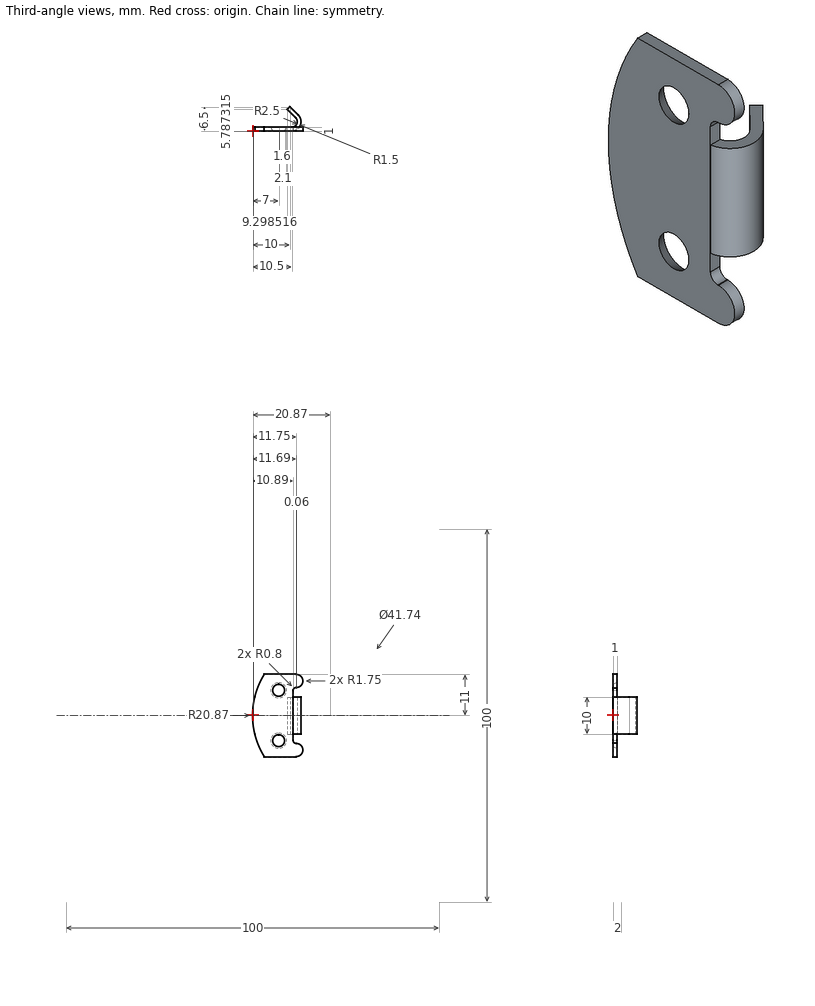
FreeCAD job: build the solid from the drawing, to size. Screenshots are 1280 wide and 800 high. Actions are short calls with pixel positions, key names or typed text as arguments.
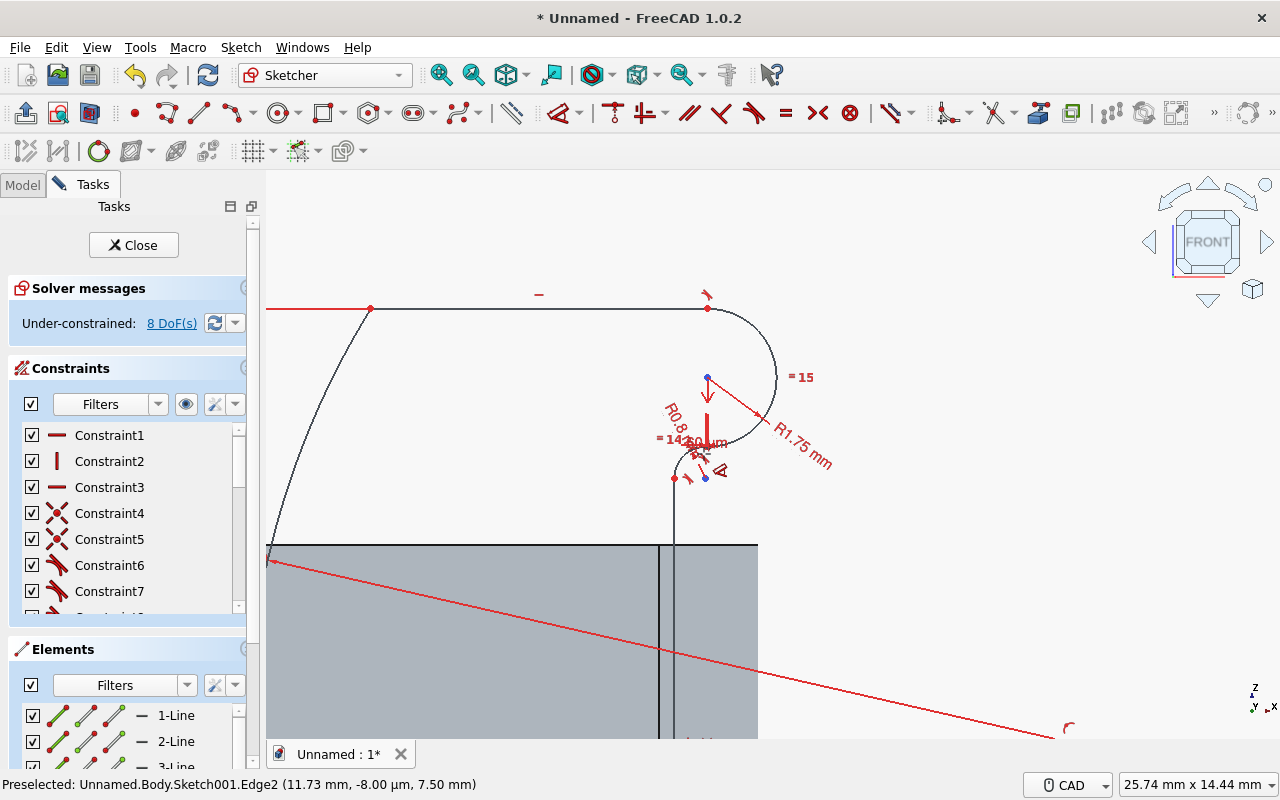
scroll(862, 220, down, 4)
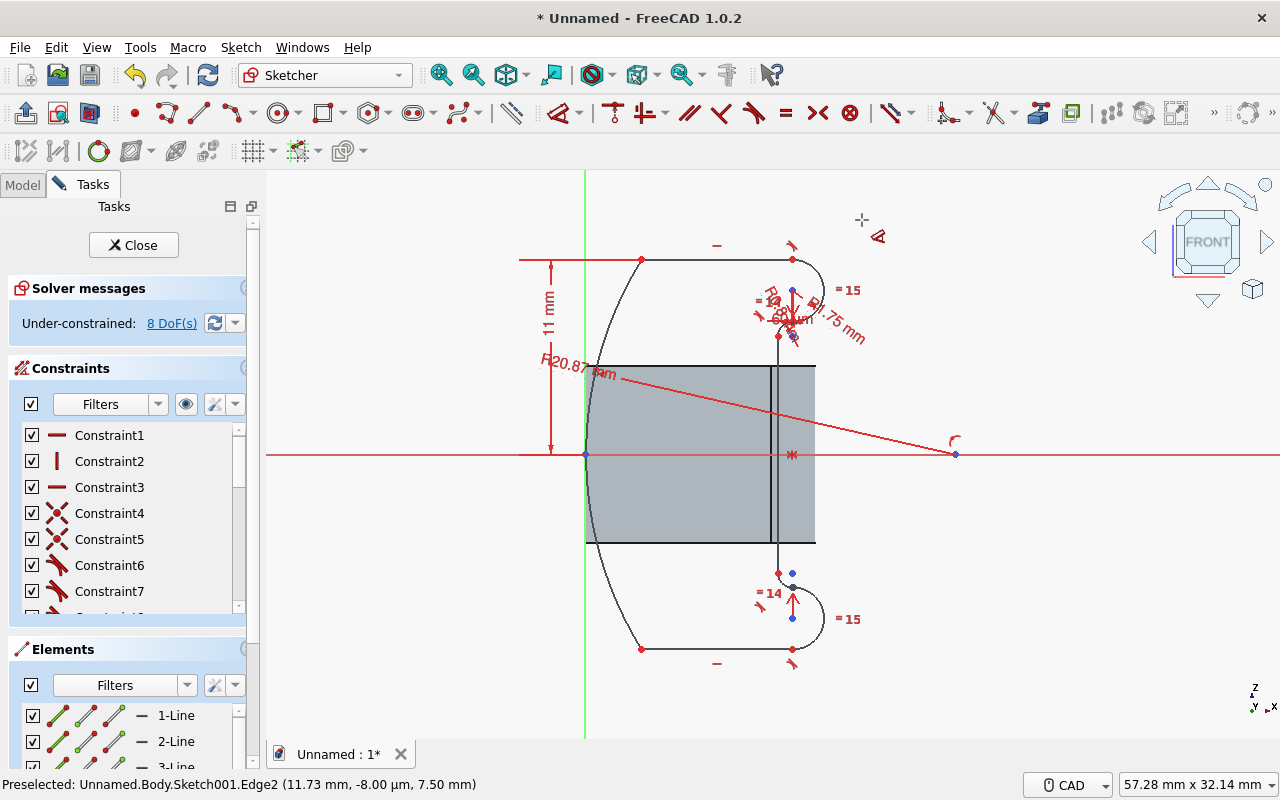
scroll(794, 587, up, 19)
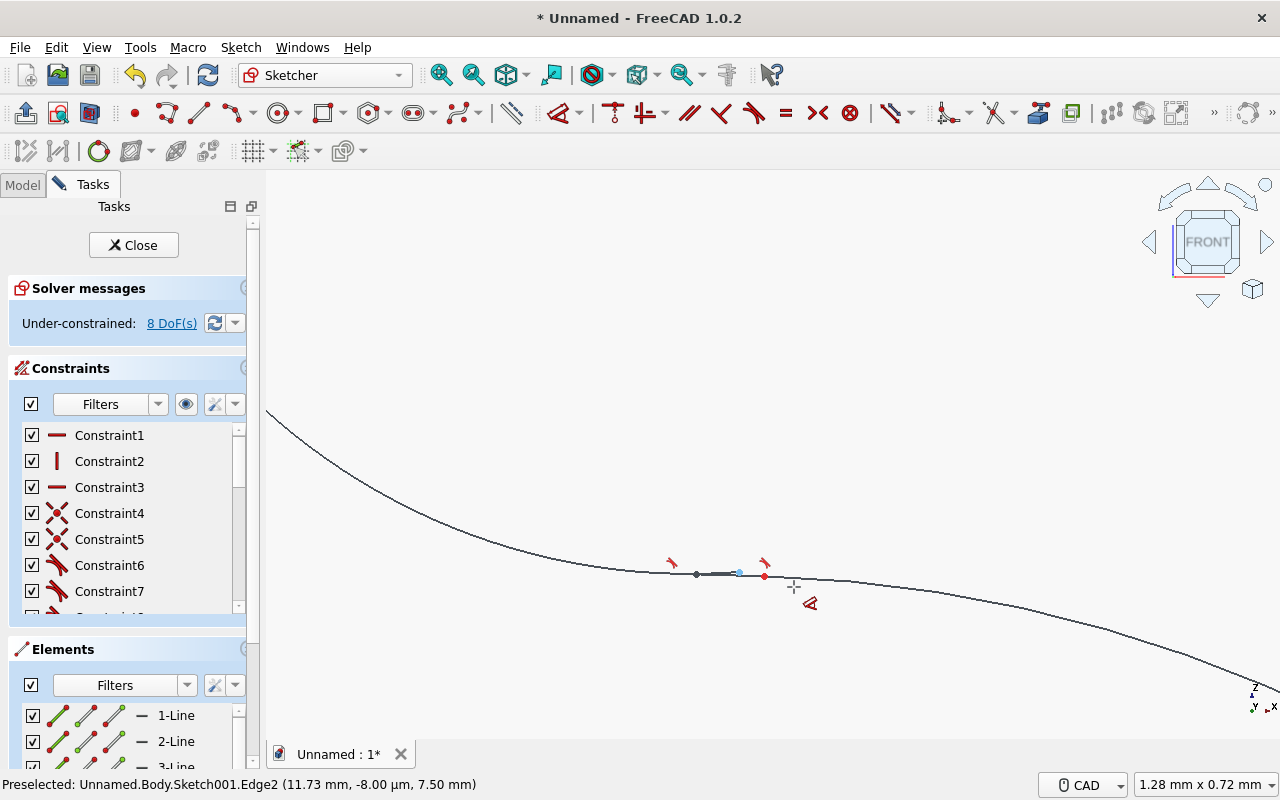
click(751, 576)
click(731, 610)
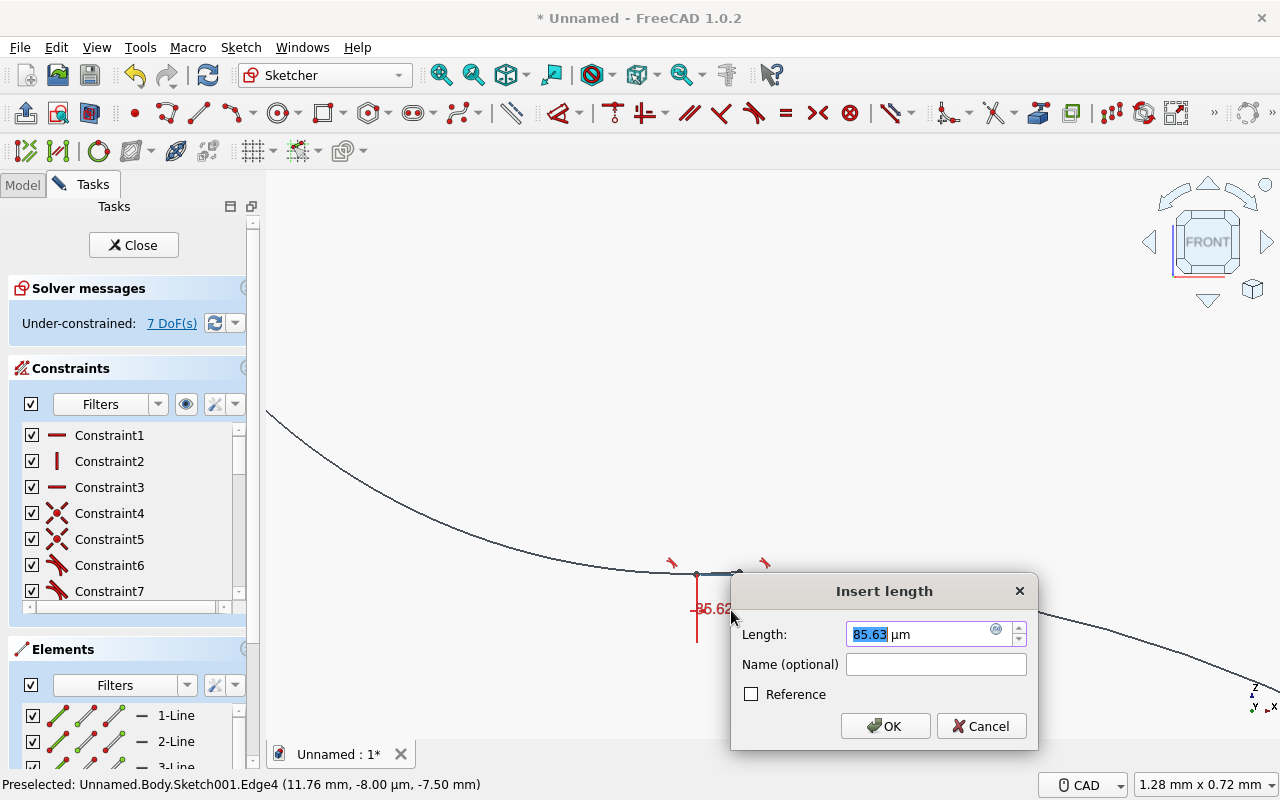
key(ctrl+a)
text(0.06 mm)
key(Return)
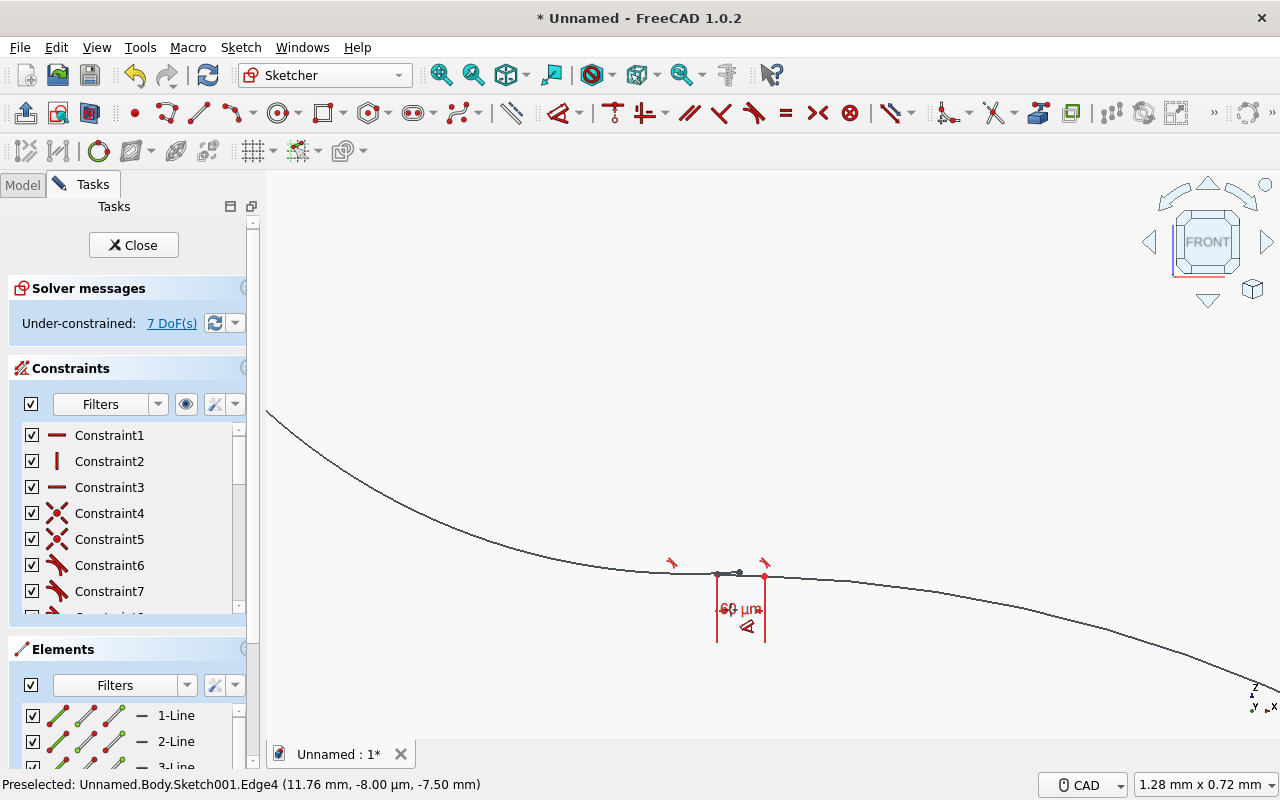
scroll(704, 454, down, 15)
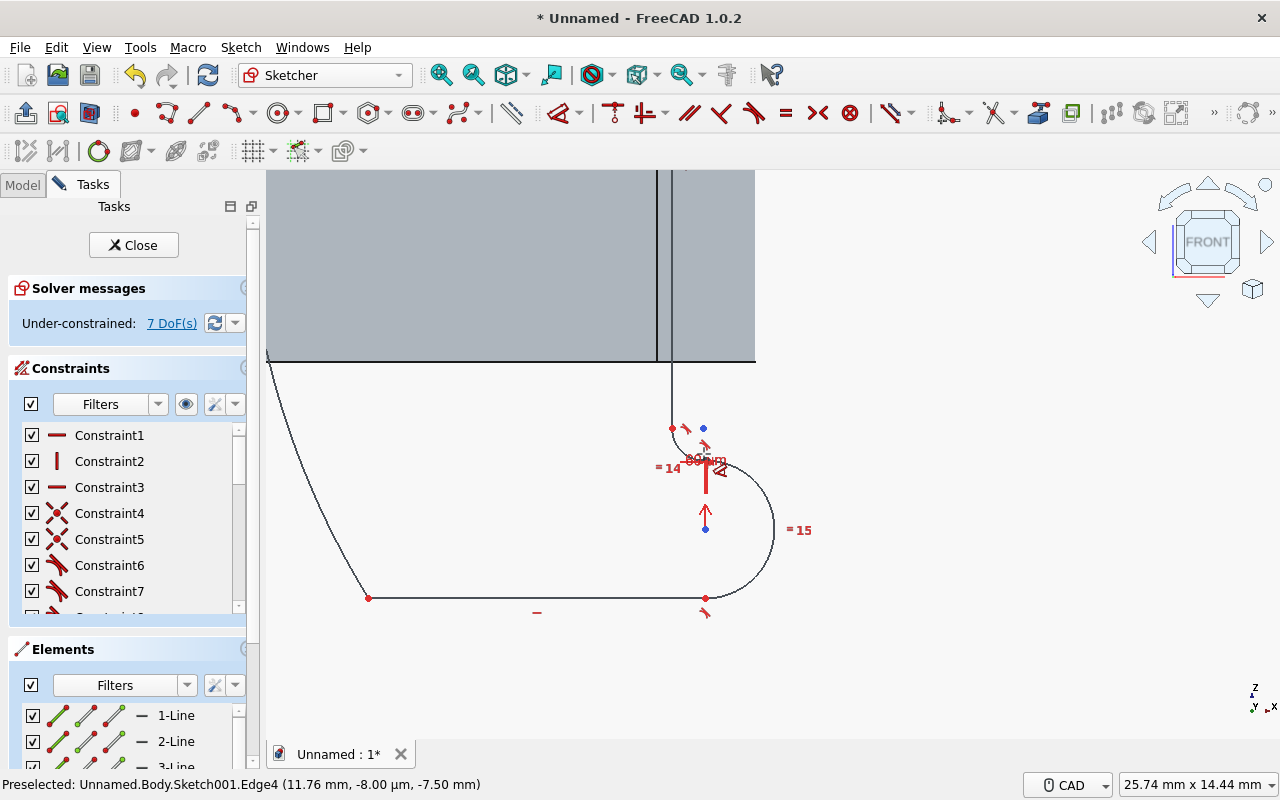
scroll(864, 691, down, 4)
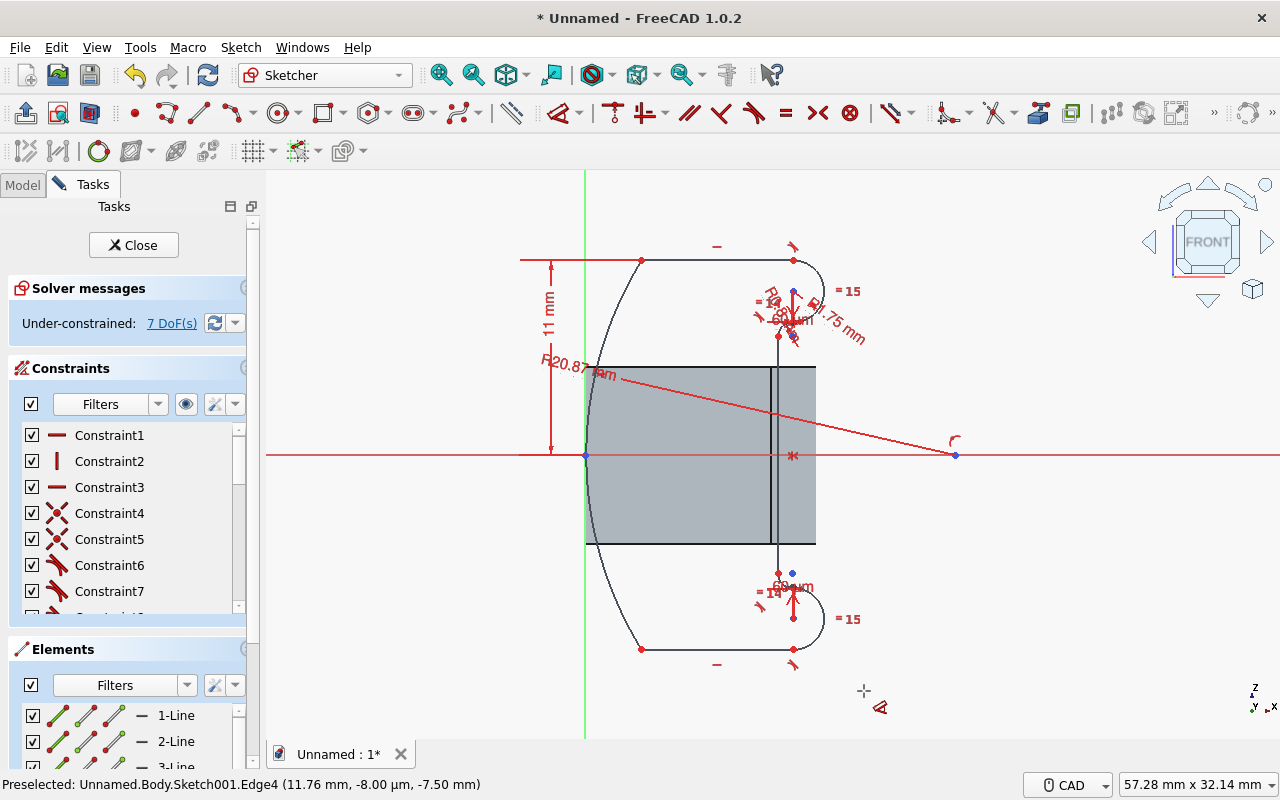
click(793, 260)
click(689, 226)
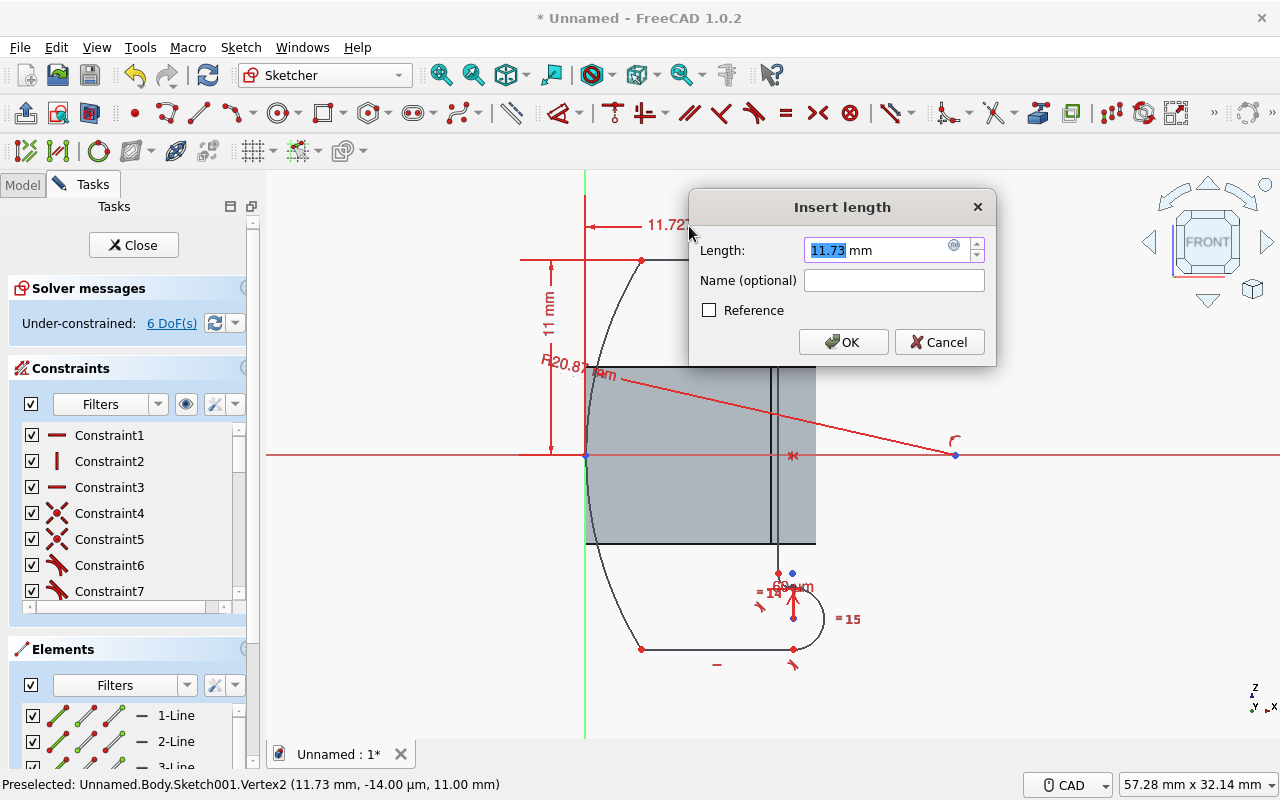
text(11.75)
key(Return)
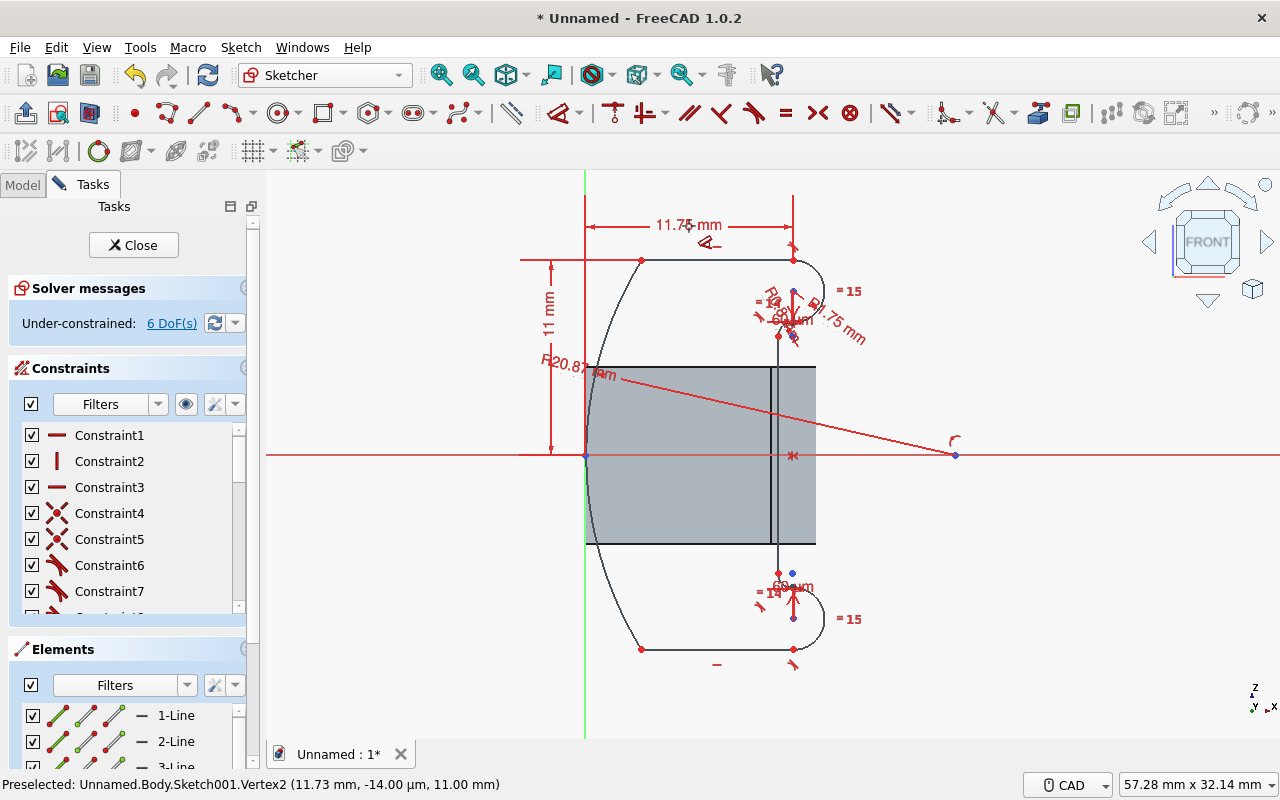
scroll(793, 322, up, 13)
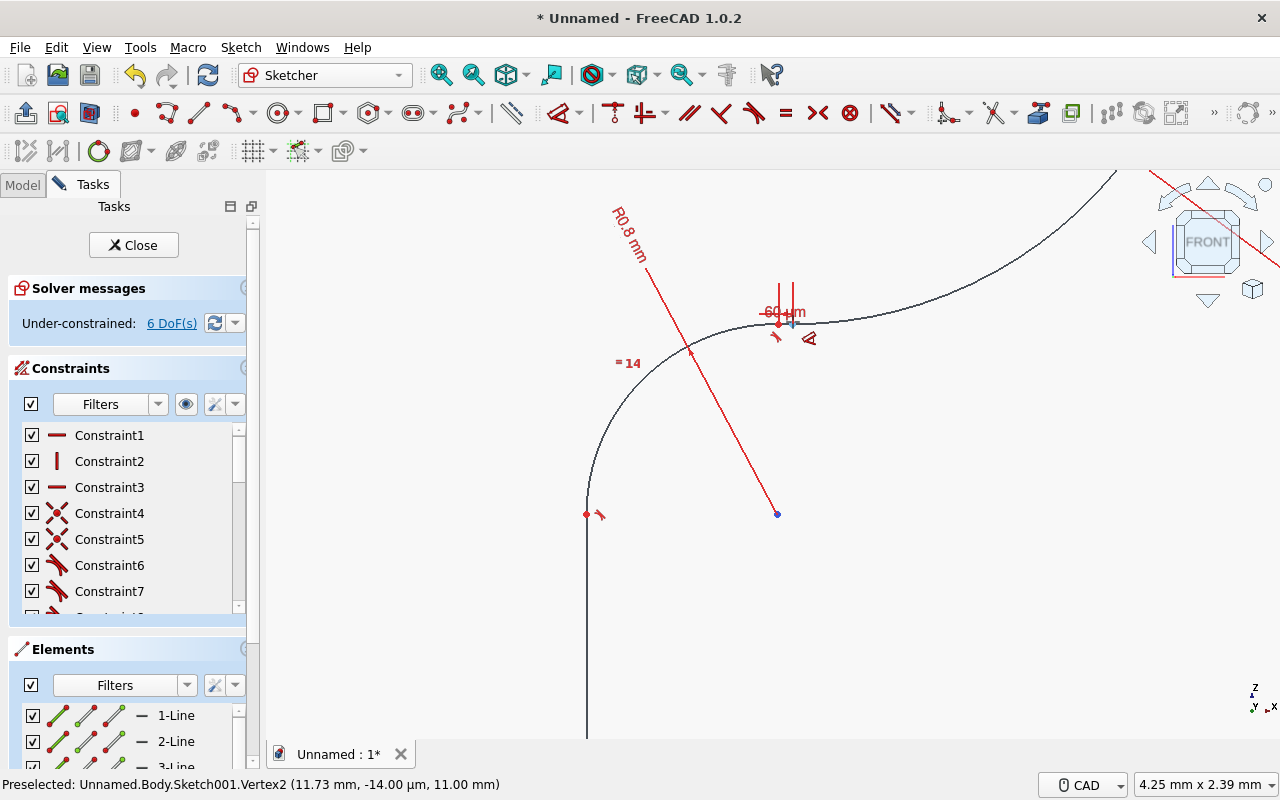
click(793, 324)
click(543, 290)